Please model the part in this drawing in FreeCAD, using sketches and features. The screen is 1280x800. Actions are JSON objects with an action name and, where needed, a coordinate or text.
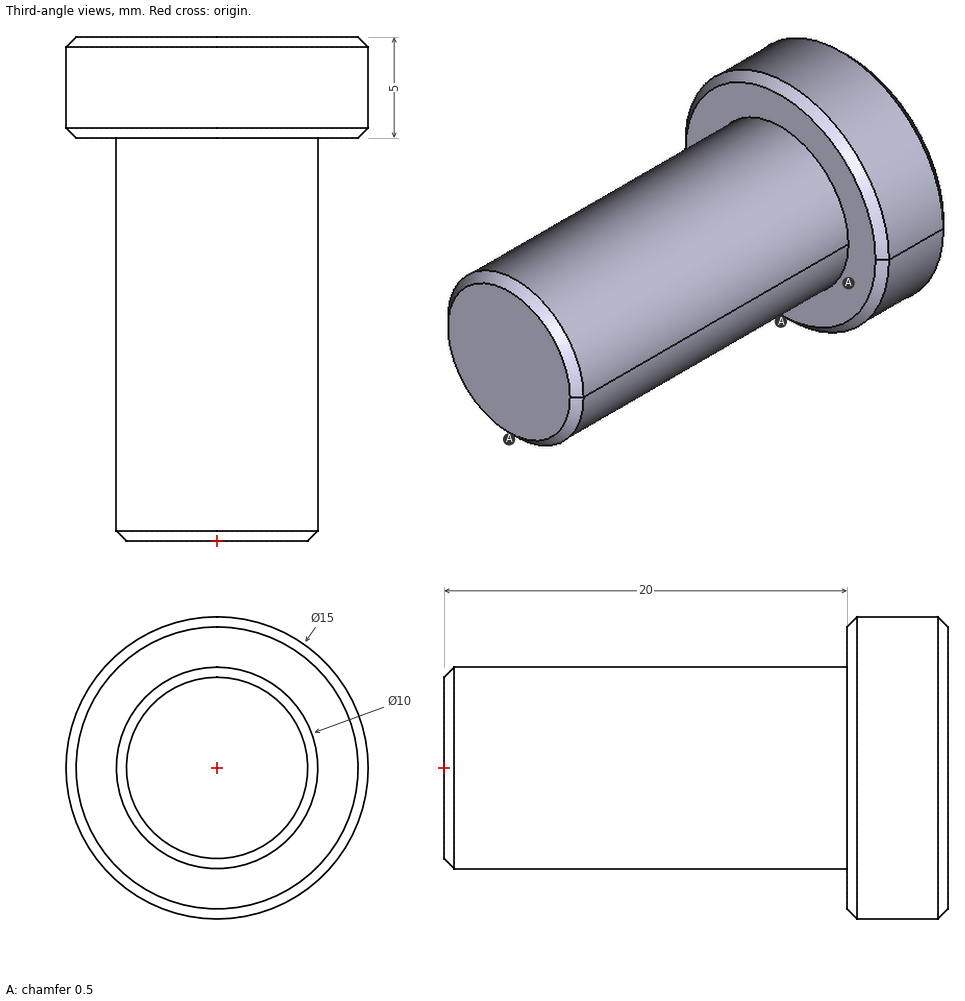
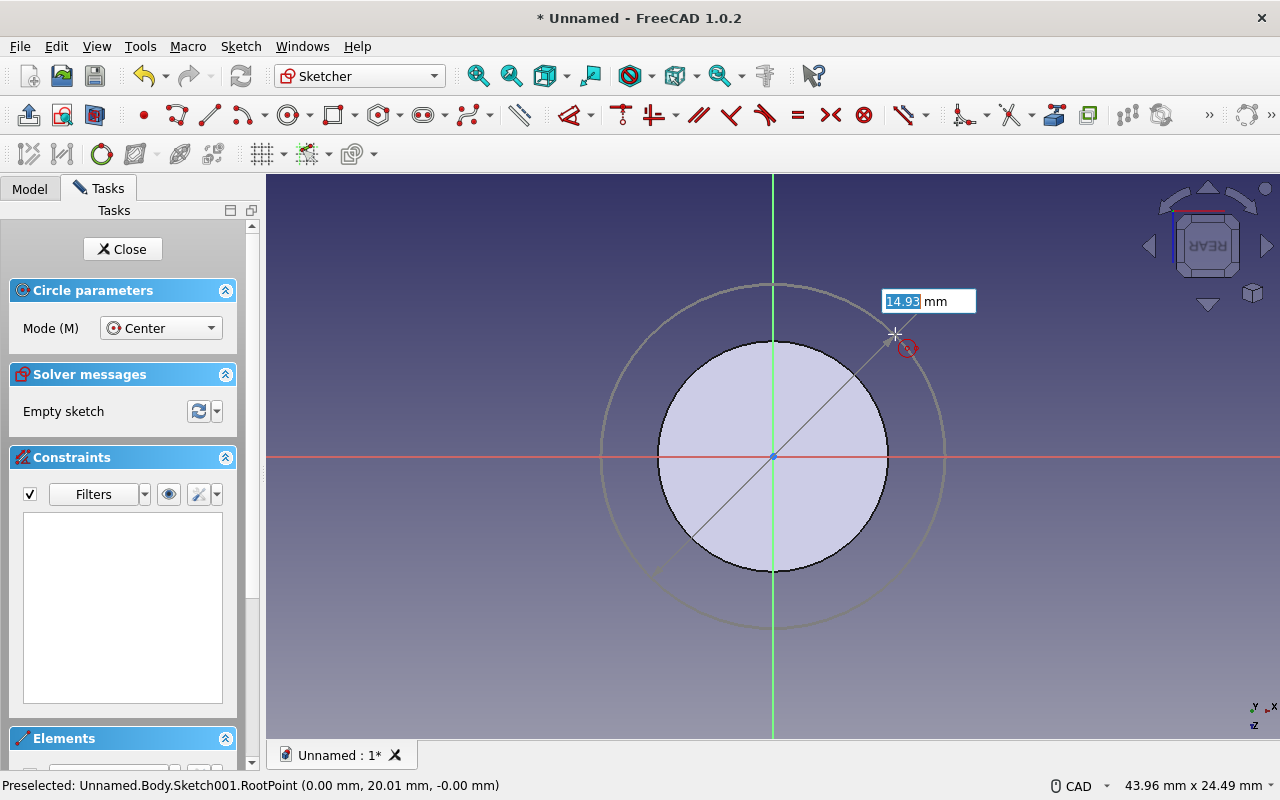
{"action": "type", "text": "15"}
{"action": "key", "text": "Return"}
{"action": "key", "text": "Escape"}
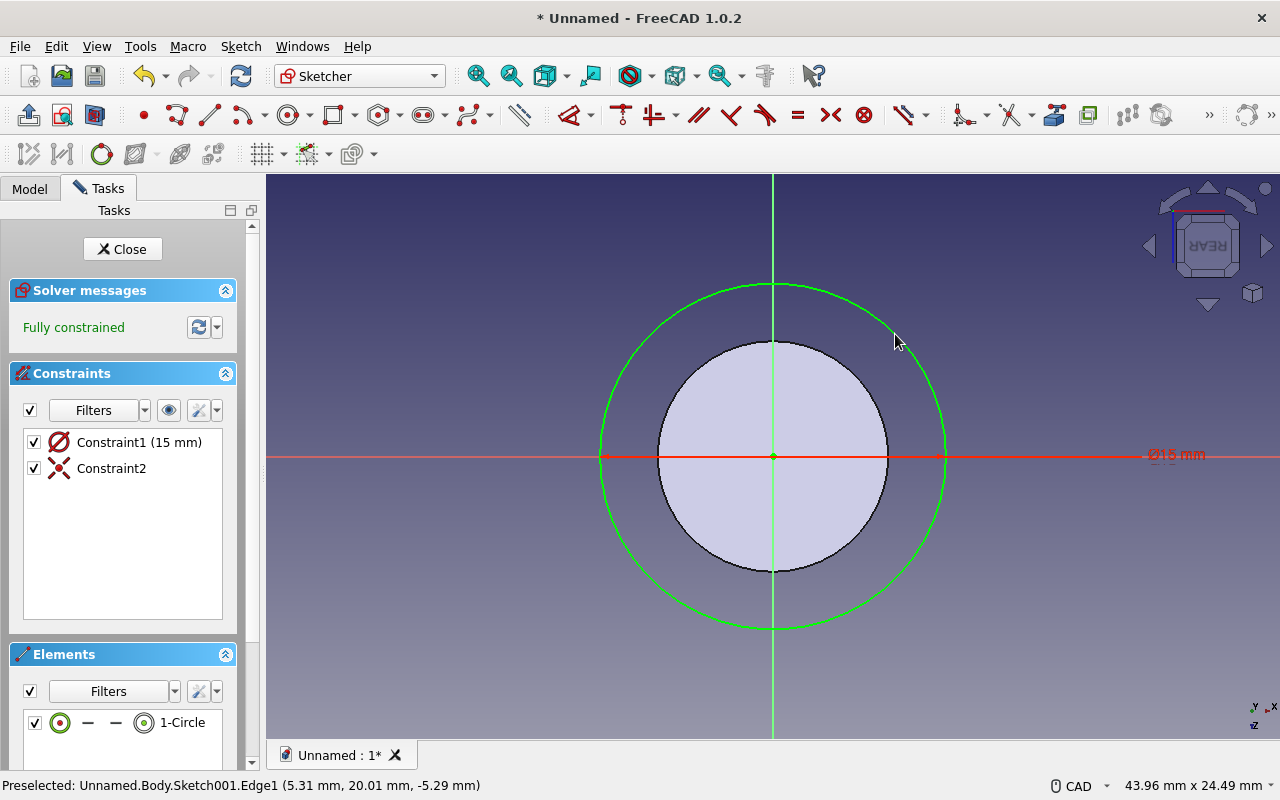
{"action": "left_click", "coordinate": [123, 249]}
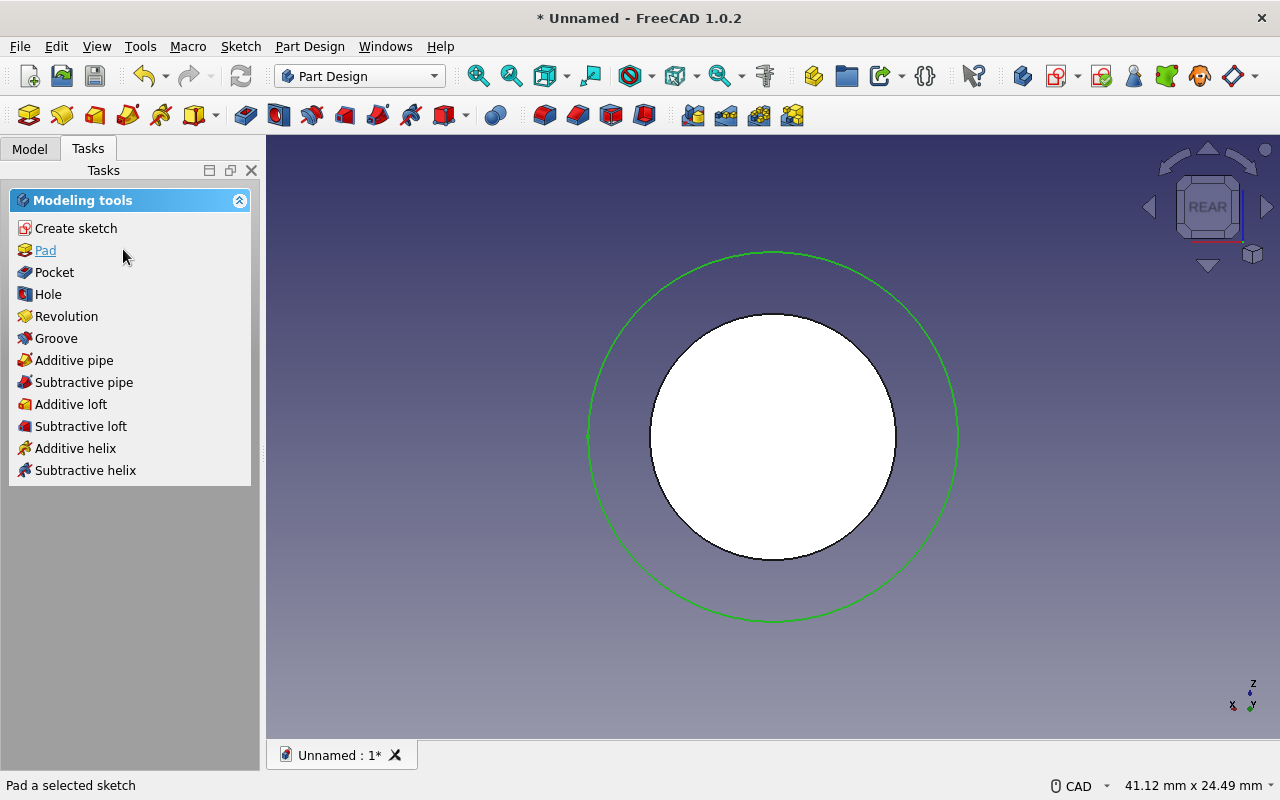
{"action": "left_click", "coordinate": [29, 116]}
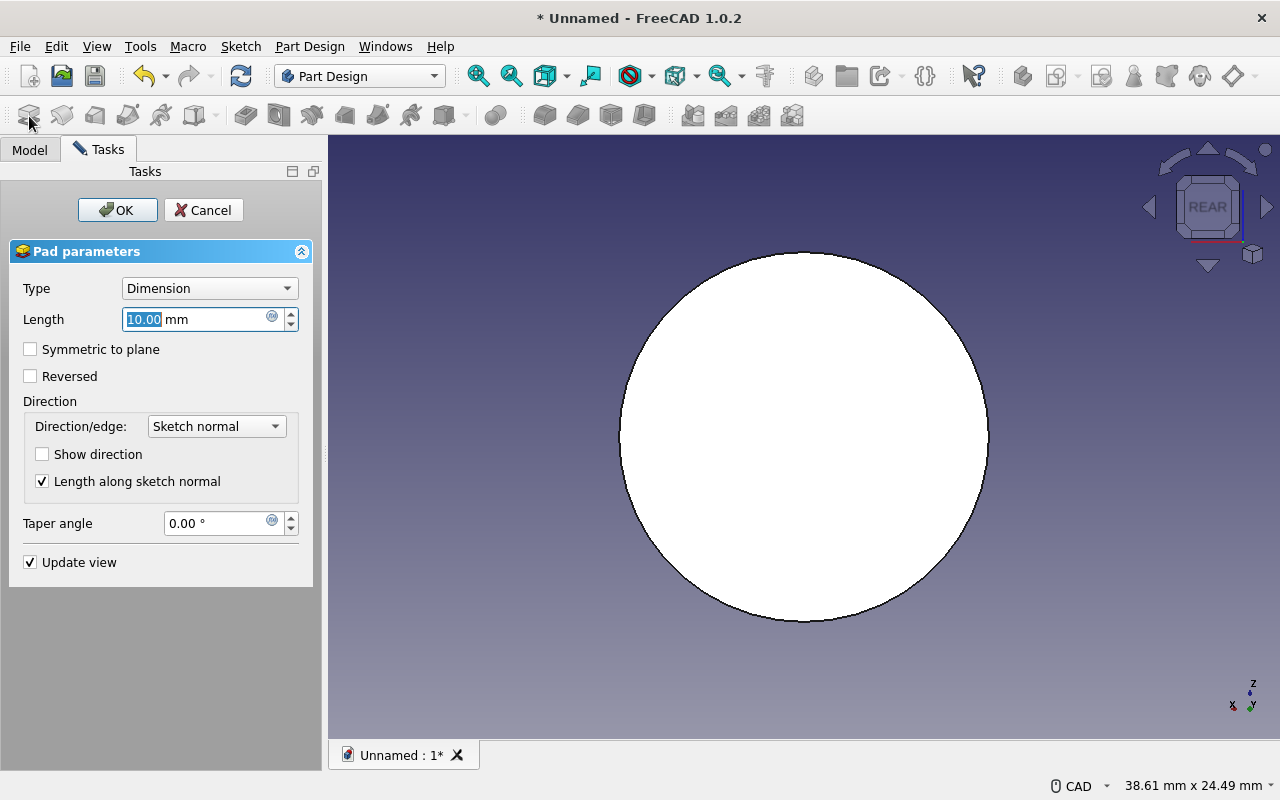
{"action": "type", "text": "5"}
{"action": "key", "text": "Tab"}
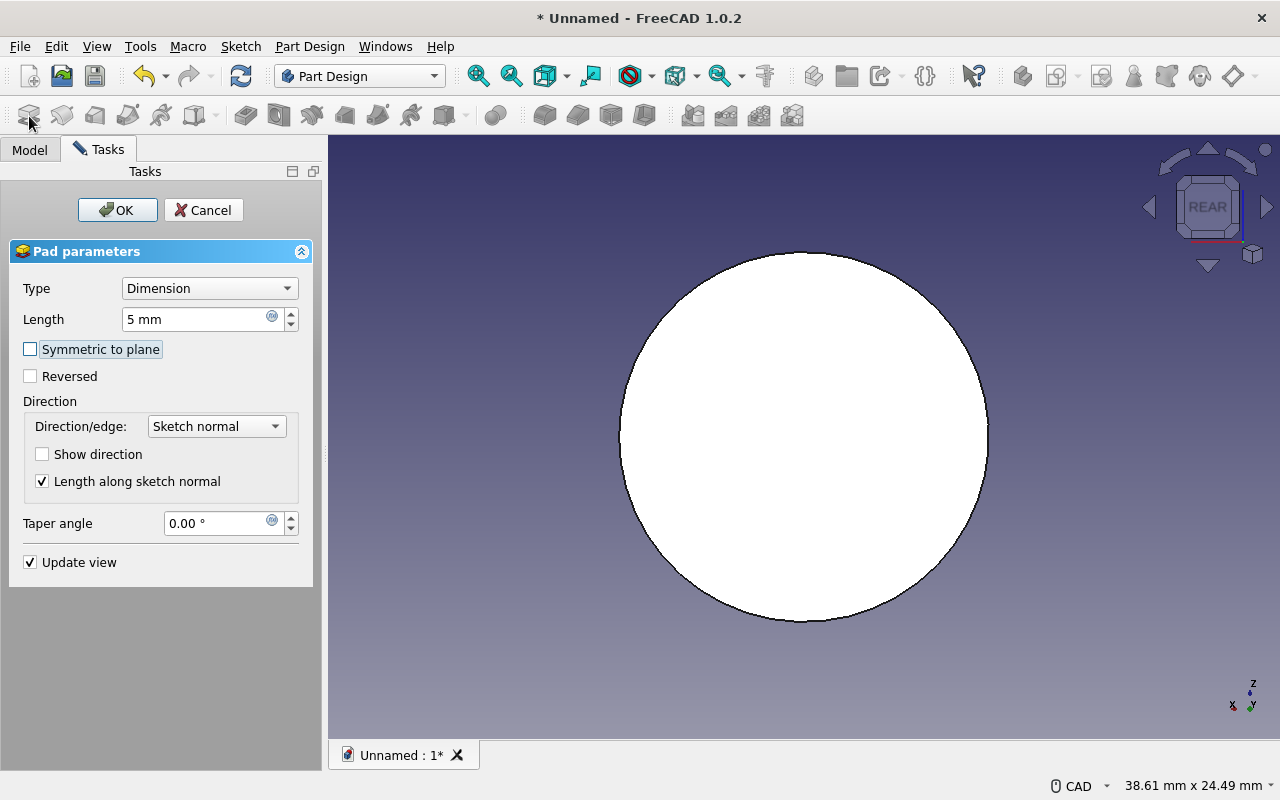
{"action": "left_click", "coordinate": [118, 210]}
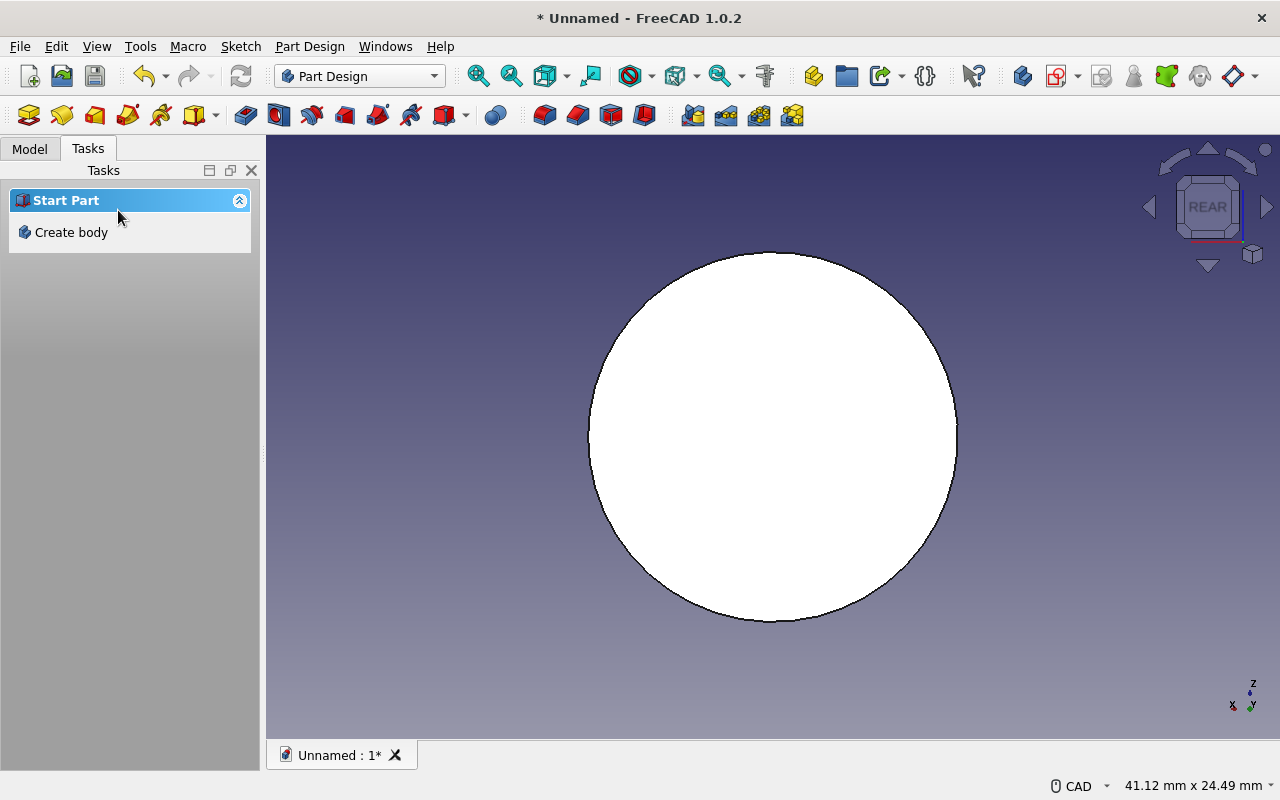
{"action": "left_click", "coordinate": [958, 436]}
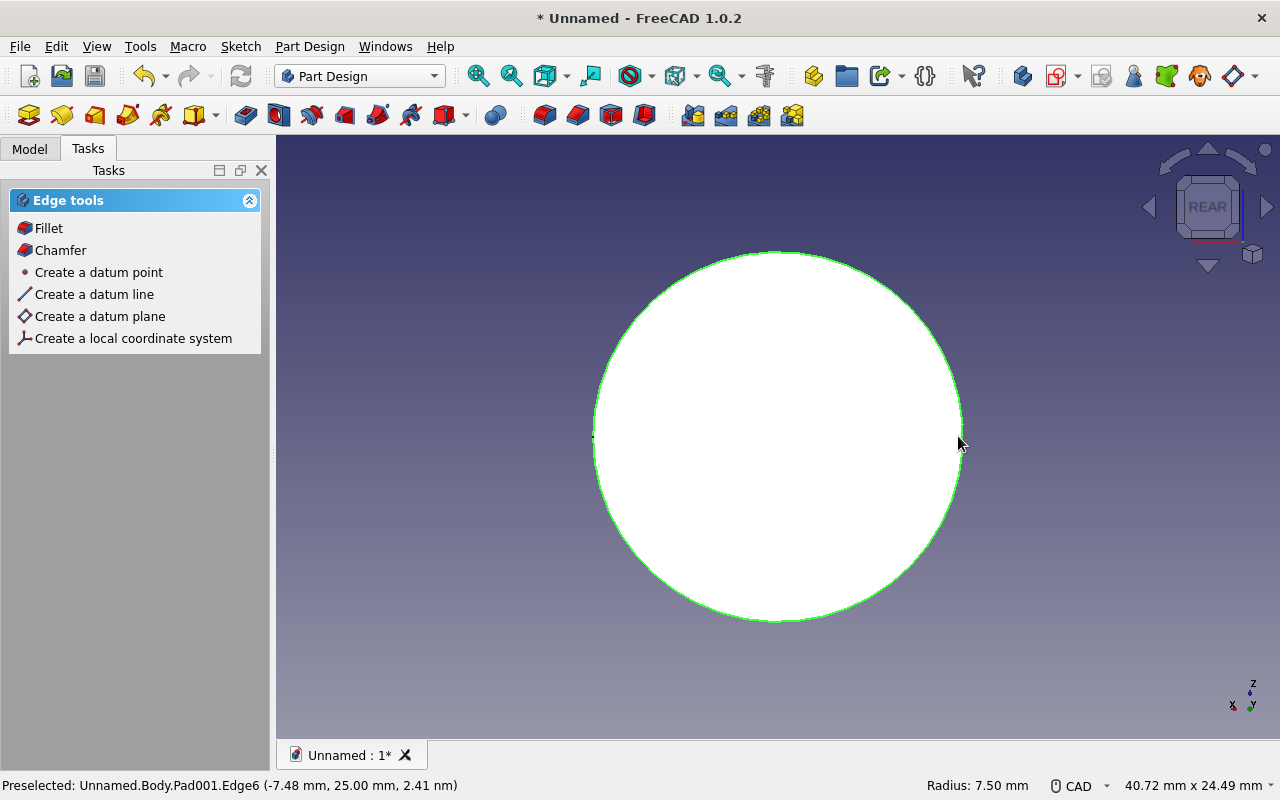
{"action": "key", "text": "0"}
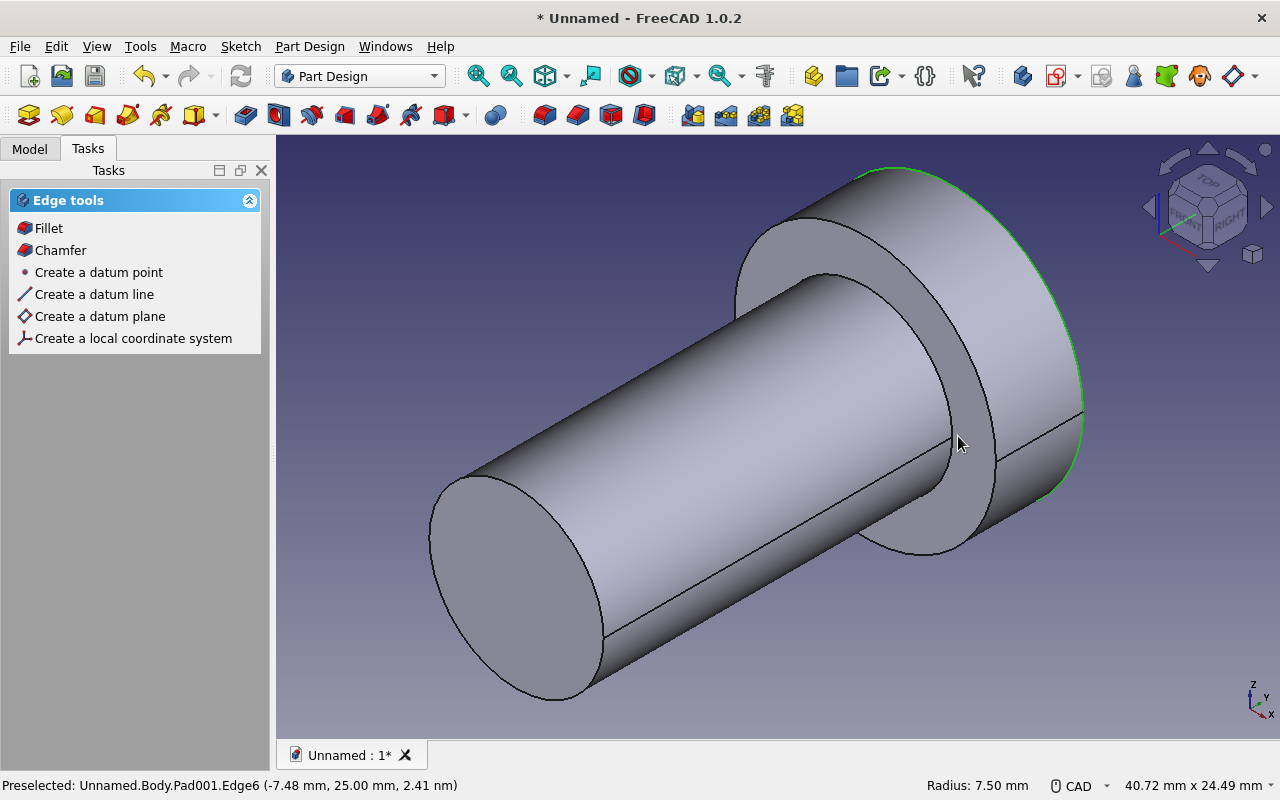
{"action": "key", "text": "v f"}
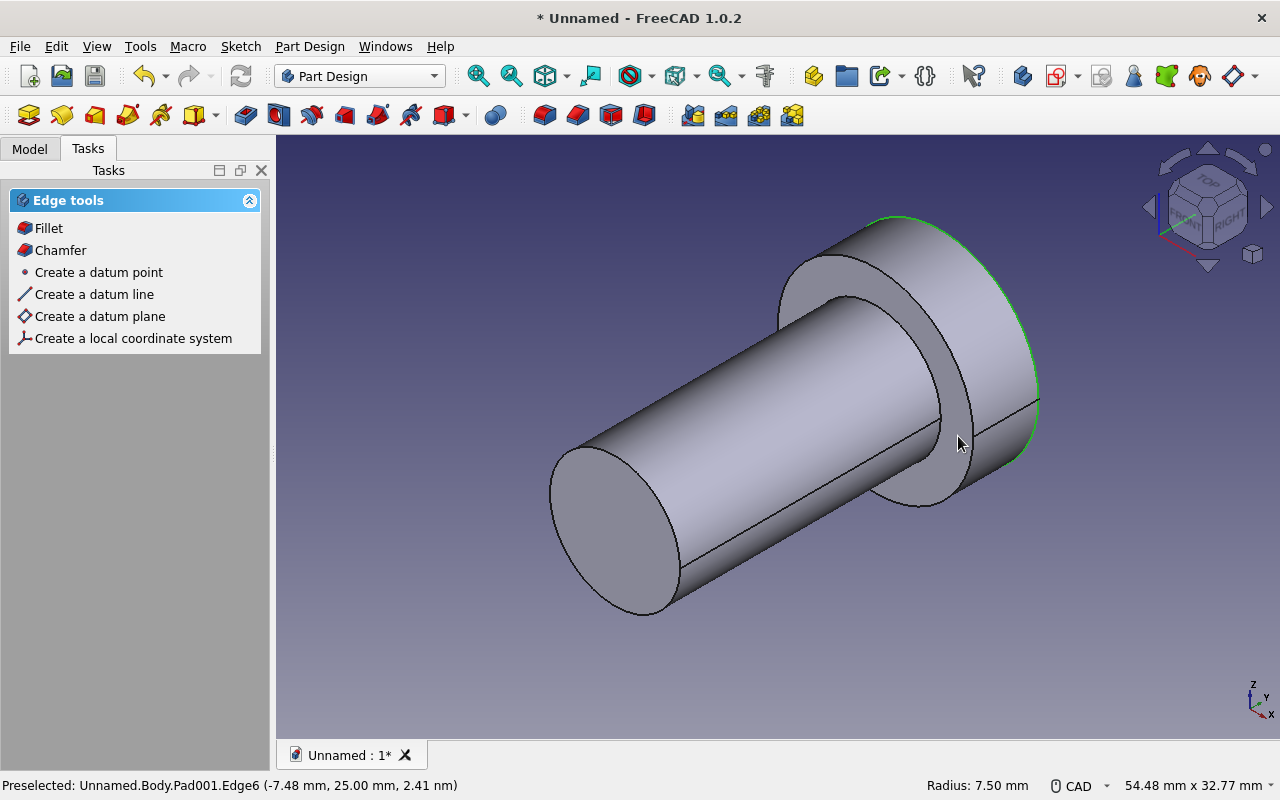
{"action": "left_click", "coordinate": [595, 447], "text": "ctrl"}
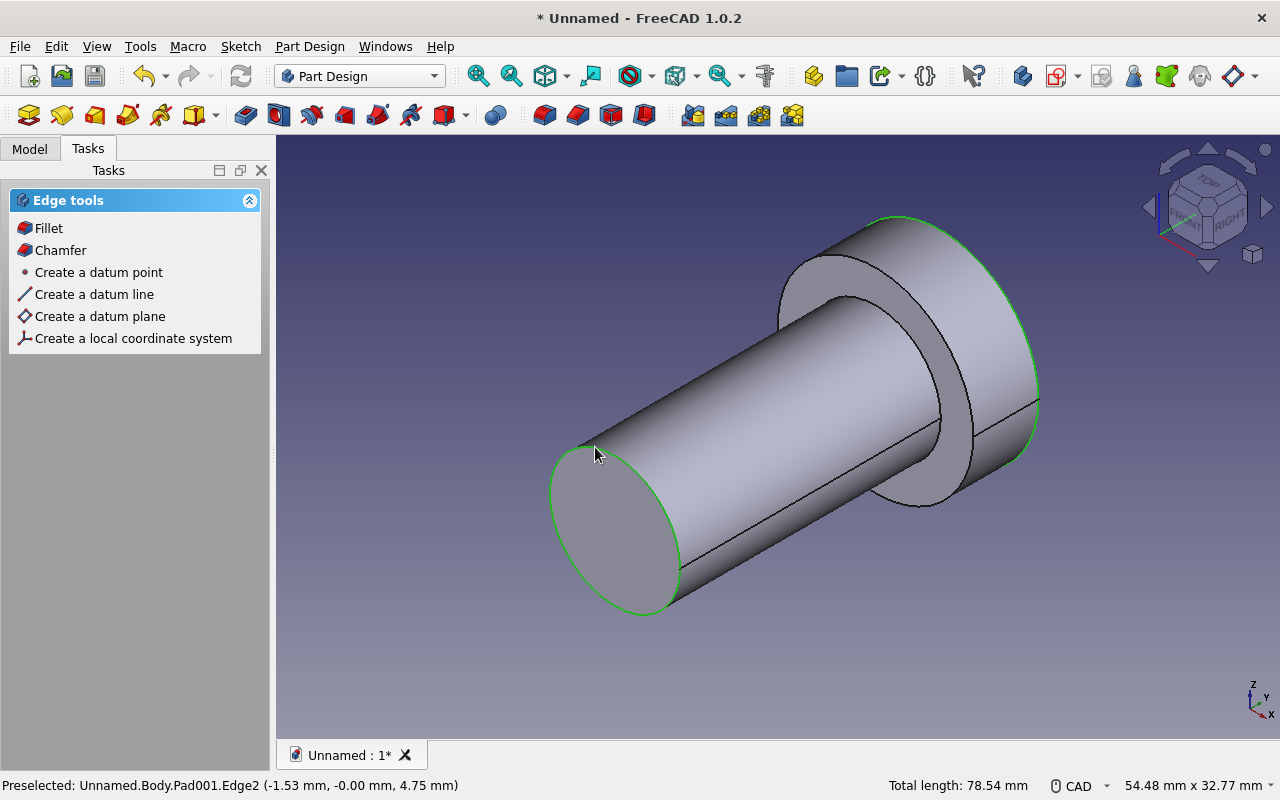
{"action": "left_click", "coordinate": [845, 255], "text": "ctrl"}